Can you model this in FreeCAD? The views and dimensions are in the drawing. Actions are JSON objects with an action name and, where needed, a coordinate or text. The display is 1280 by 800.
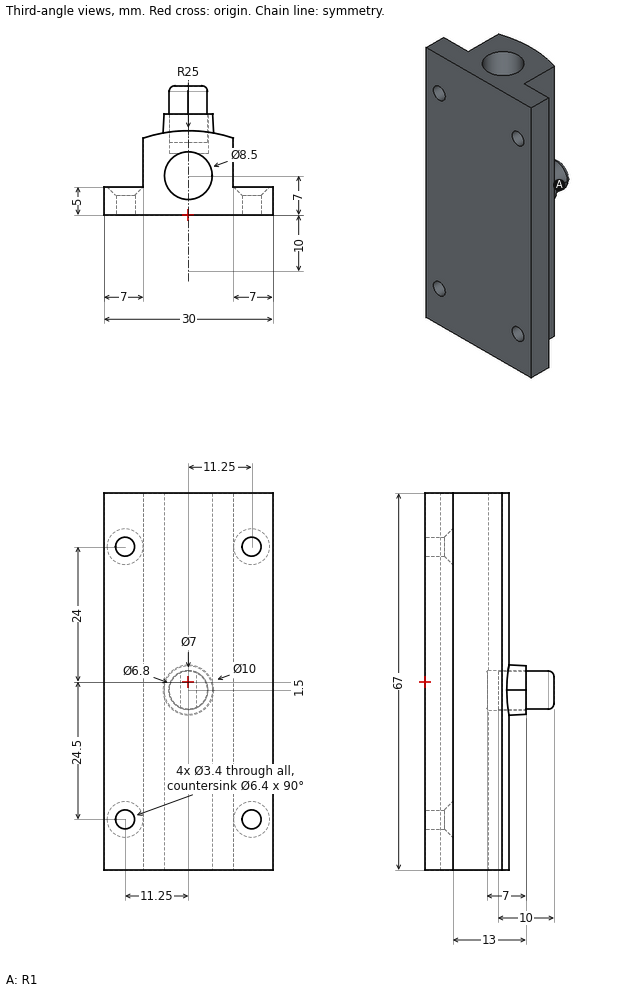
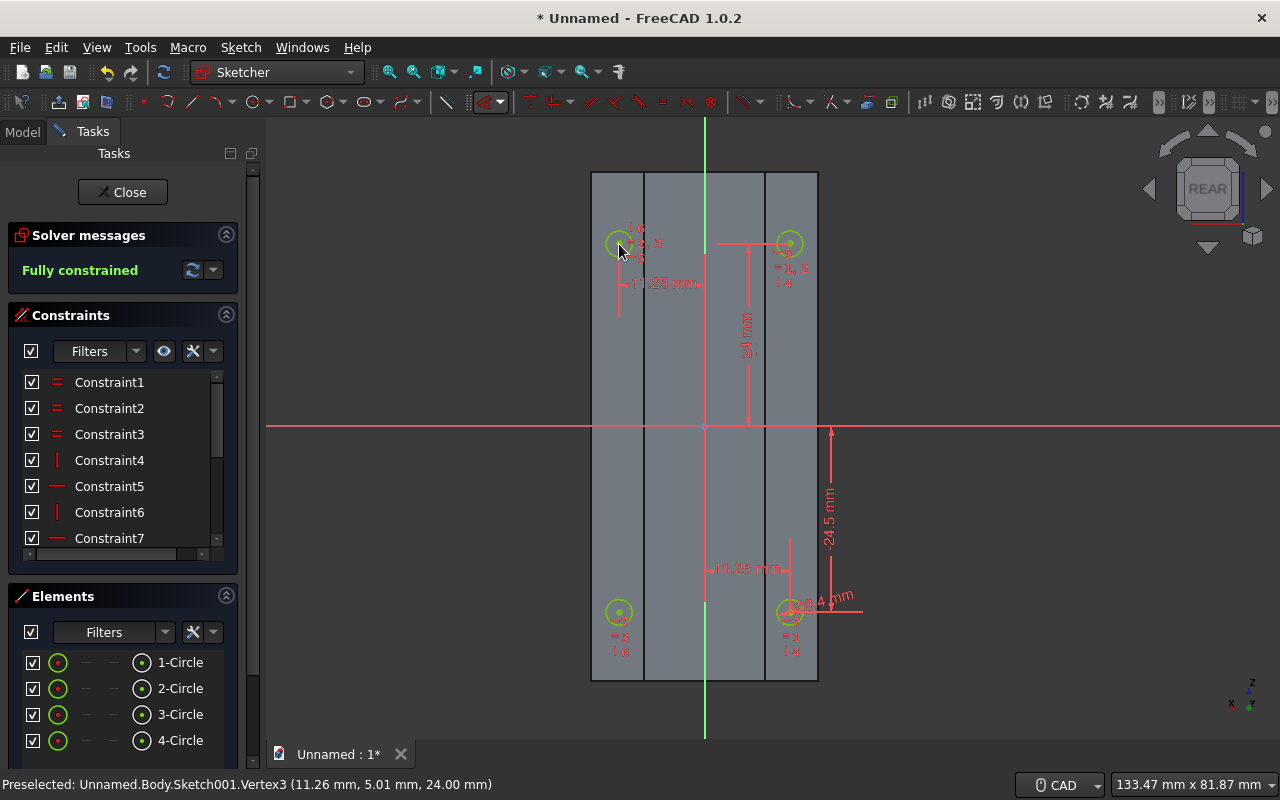
{"action": "left_click", "coordinate": [123, 192]}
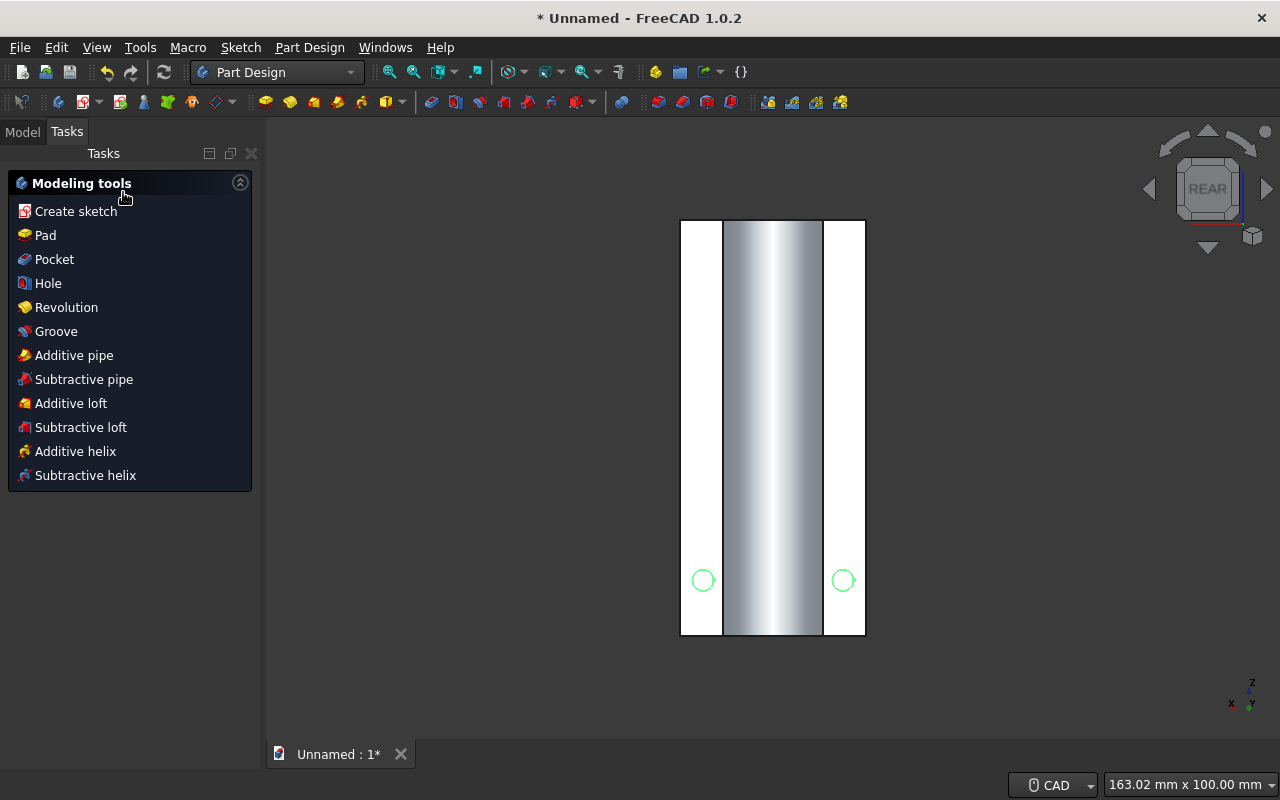
{"action": "left_click", "coordinate": [456, 102]}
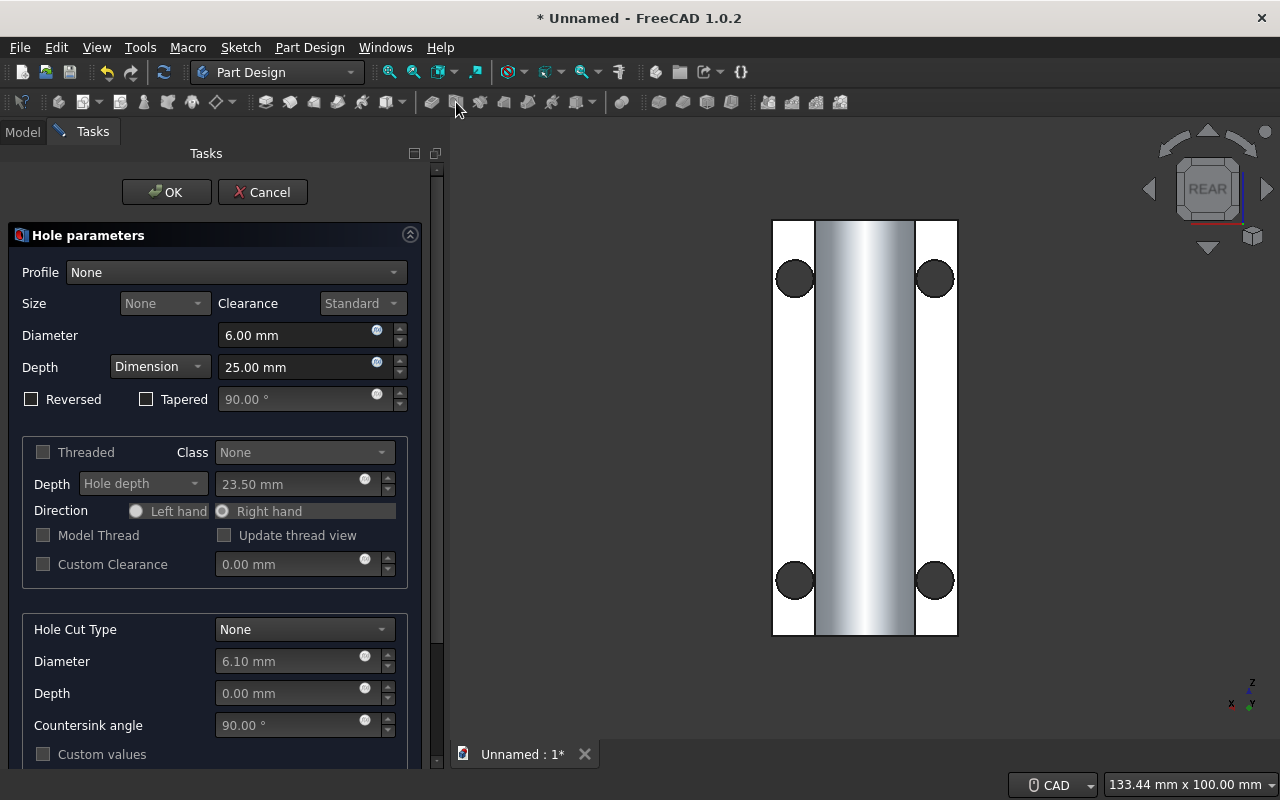
{"action": "triple_click", "coordinate": [305, 335]}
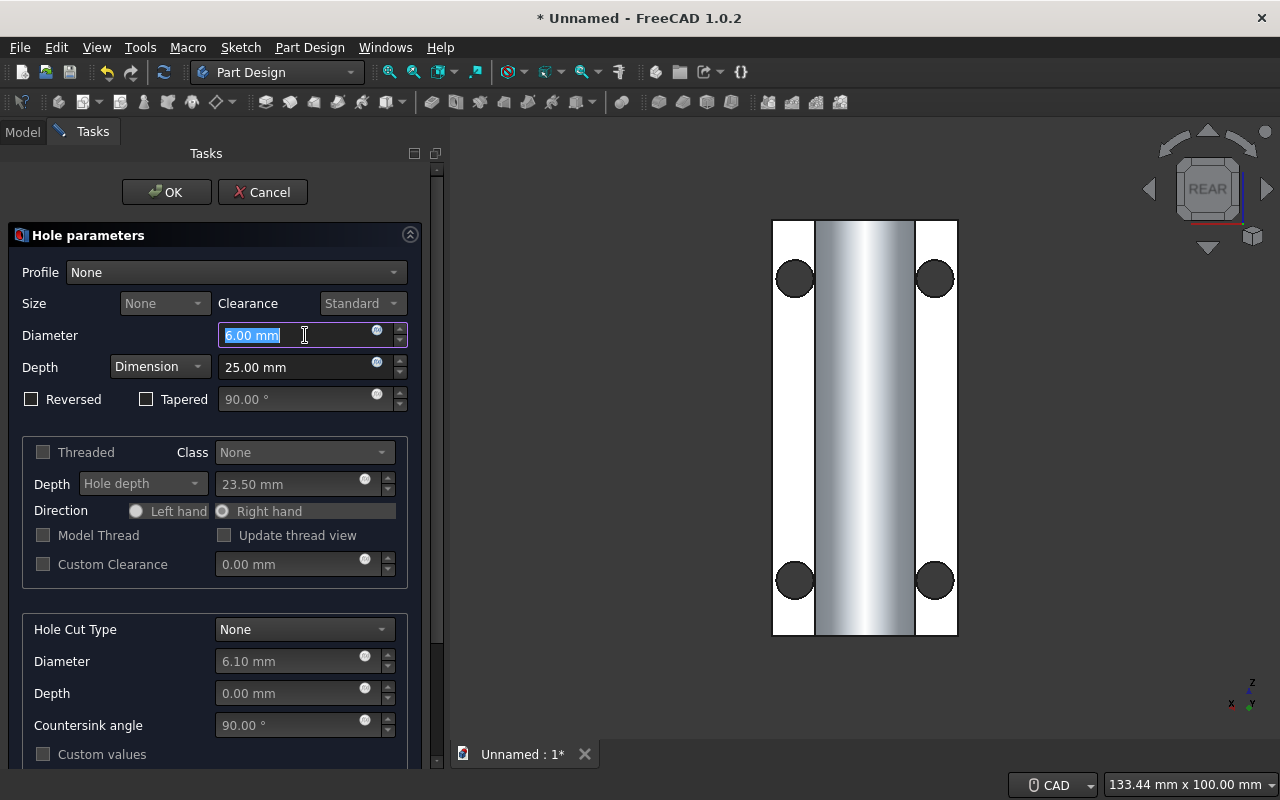
{"action": "type", "text": "3.4"}
{"action": "key", "text": "Tab"}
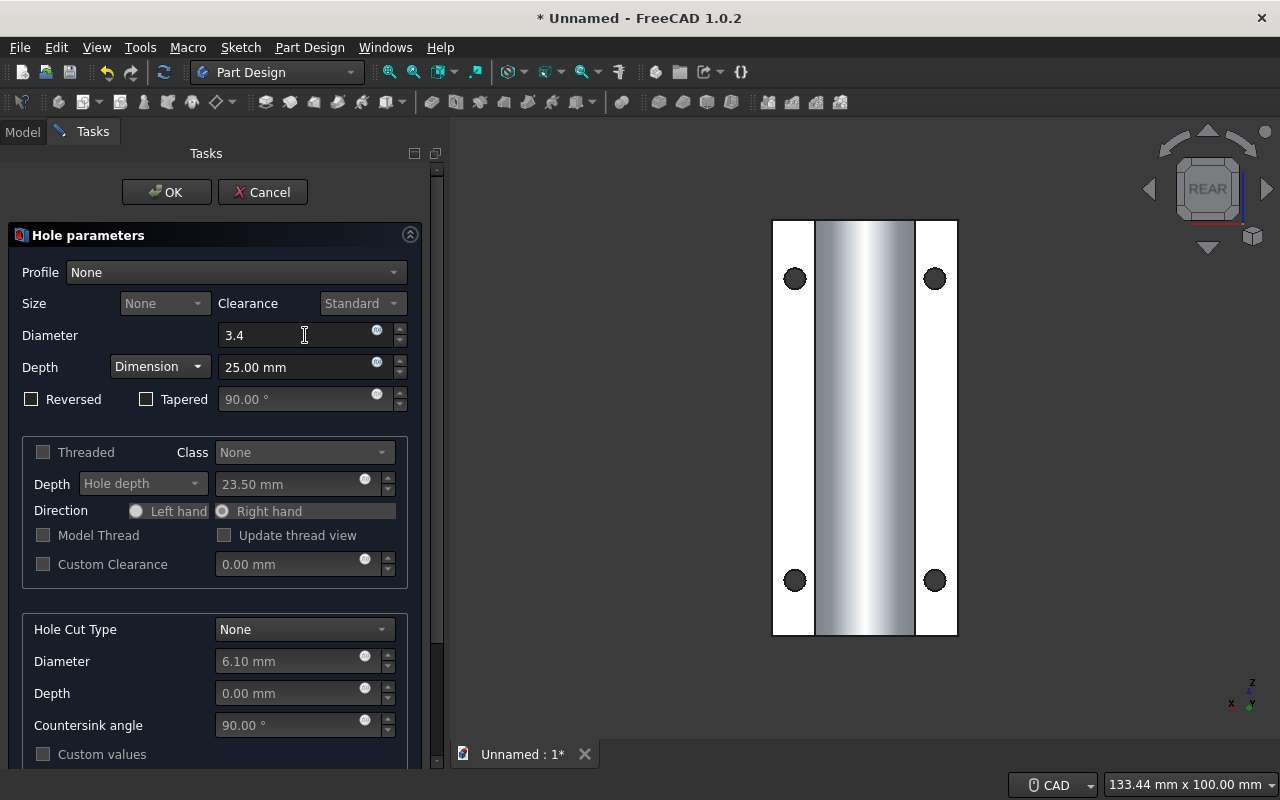
{"action": "left_click", "coordinate": [161, 366]}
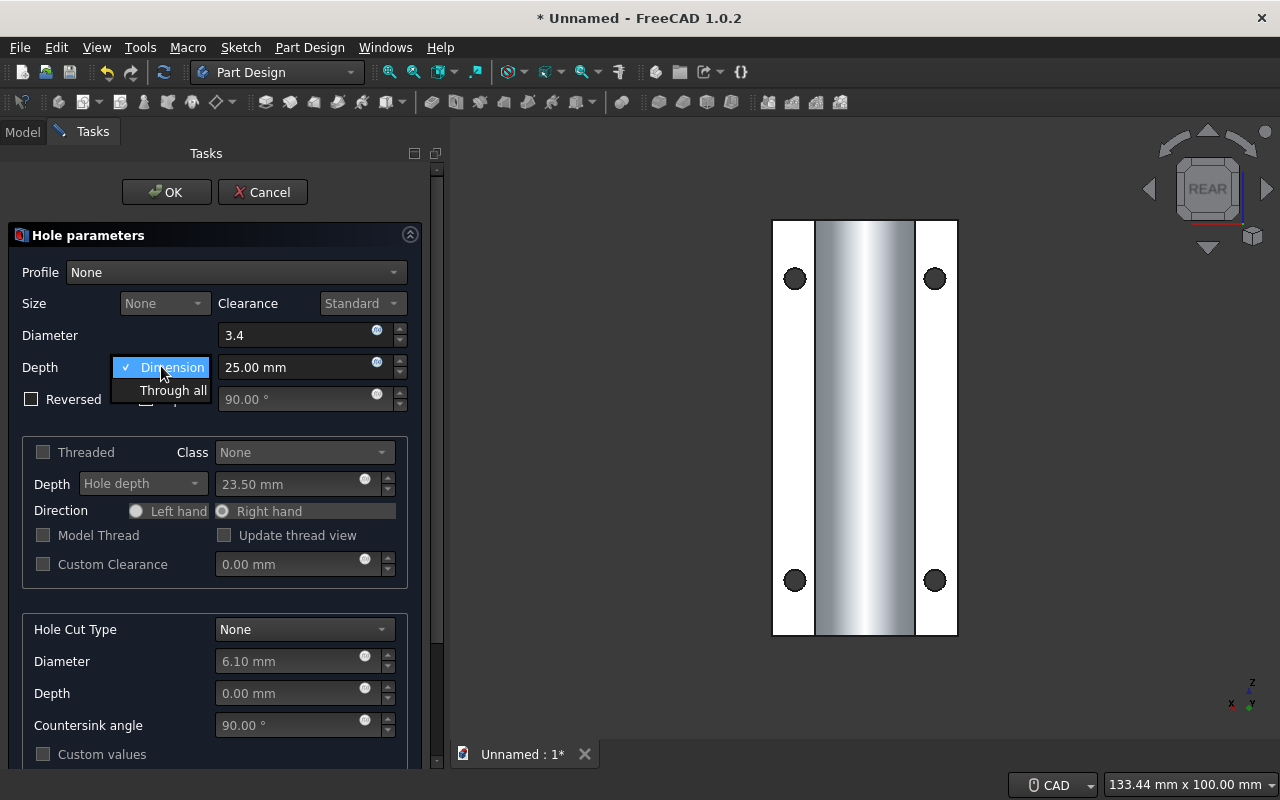
{"action": "left_click", "coordinate": [160, 390]}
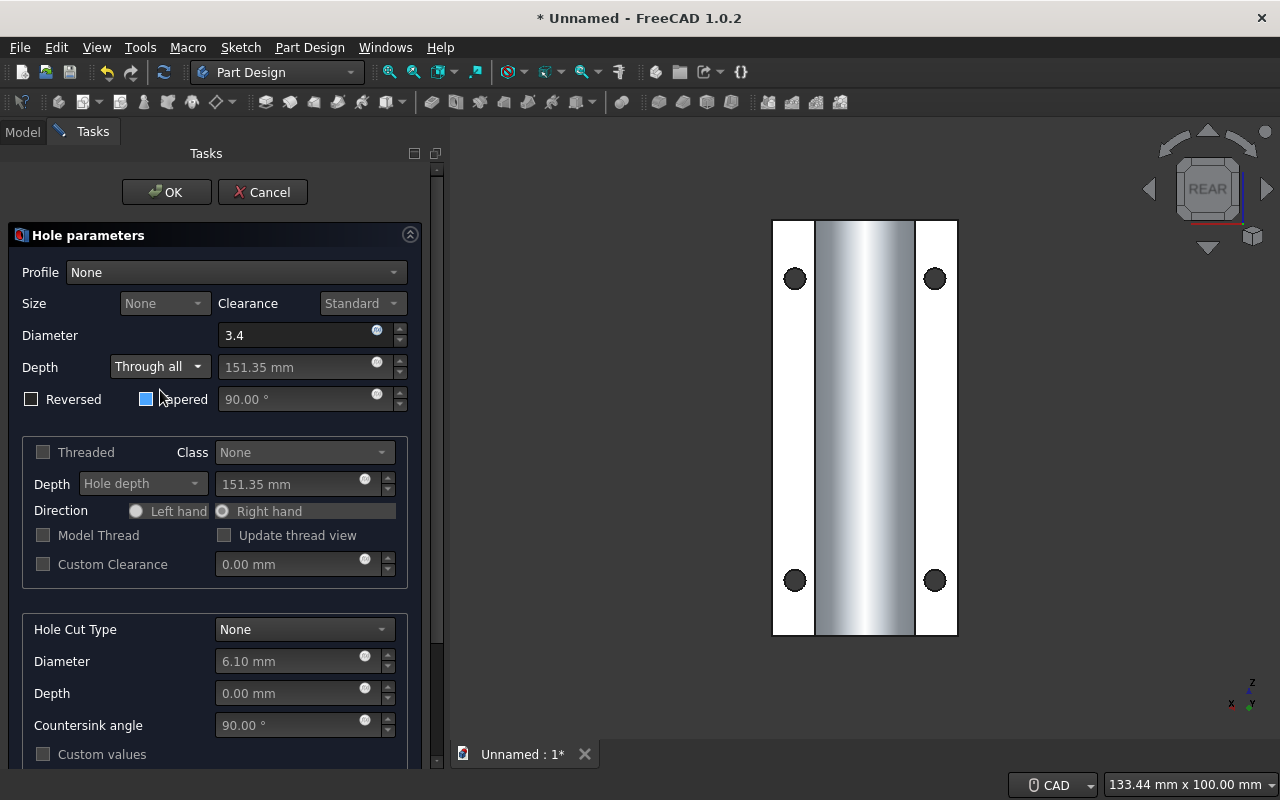
{"action": "left_click", "coordinate": [306, 630]}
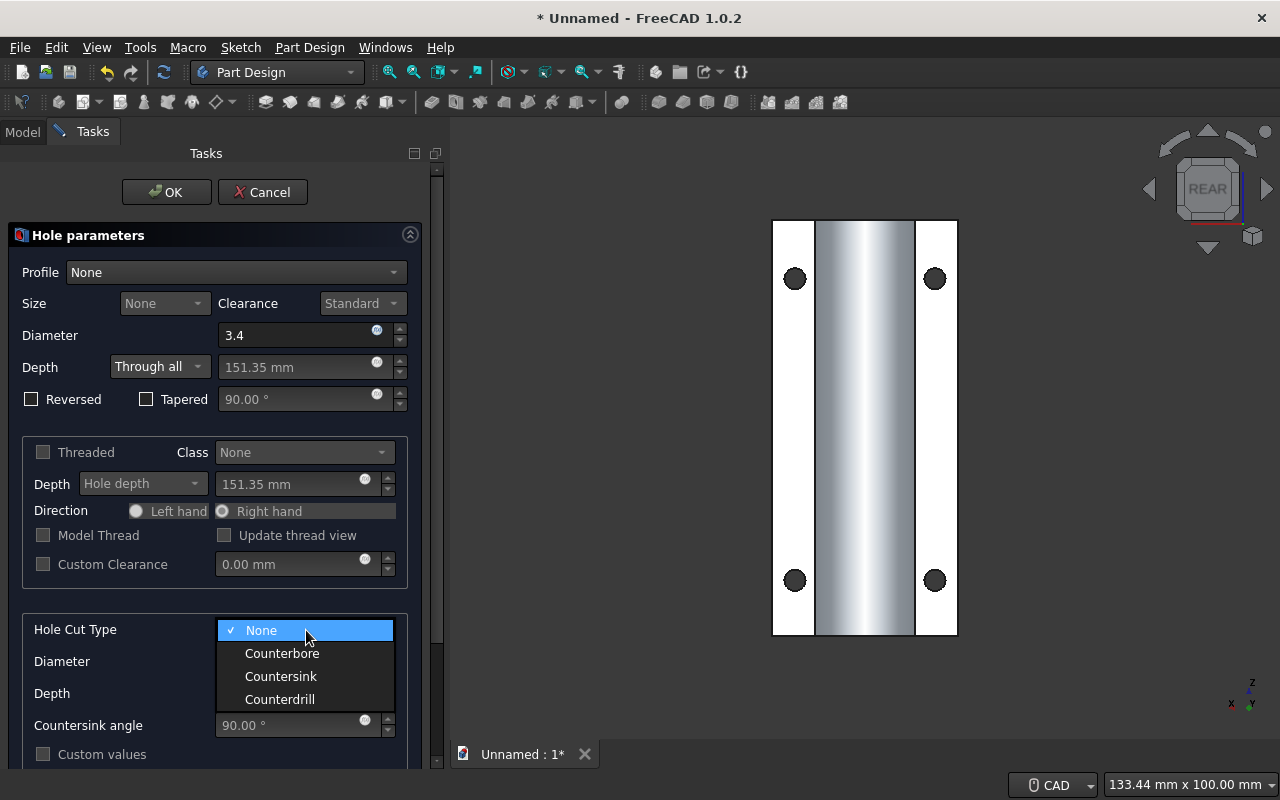
{"action": "left_click", "coordinate": [304, 676]}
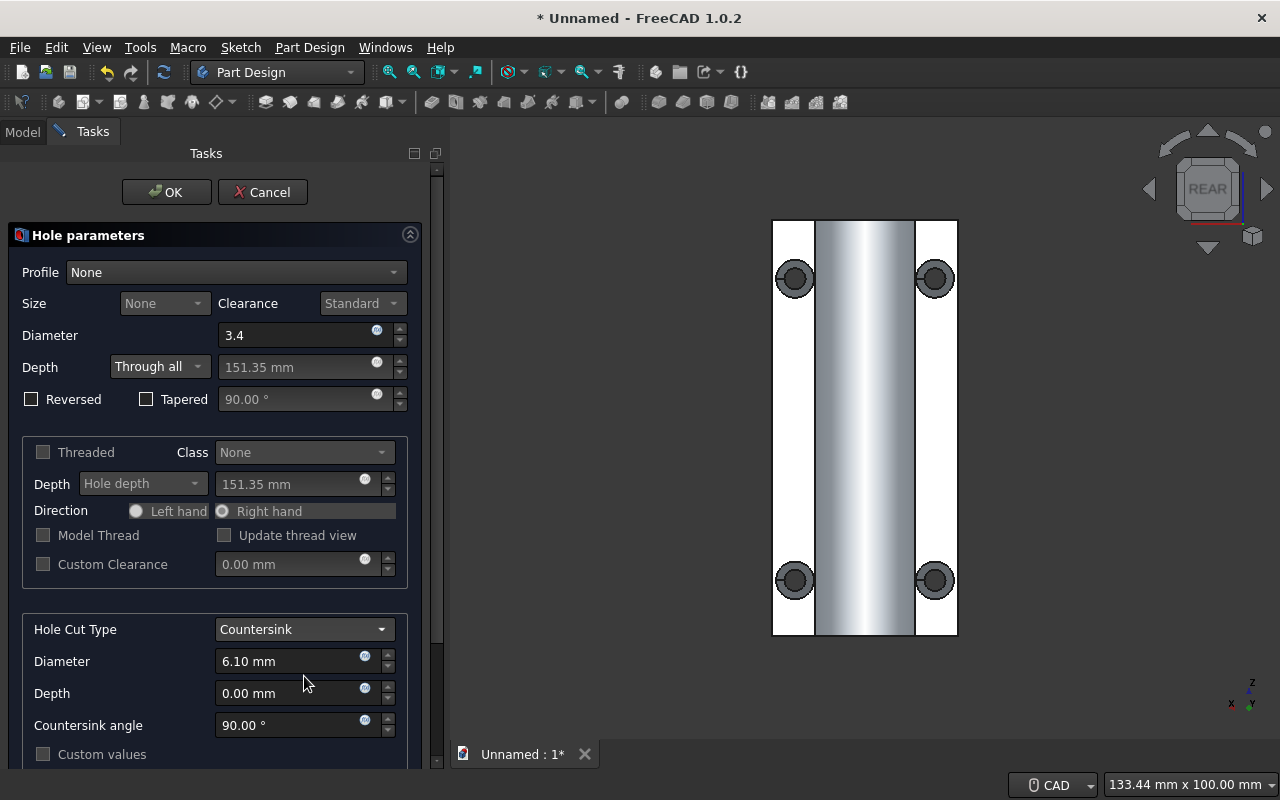
{"action": "triple_click", "coordinate": [298, 661]}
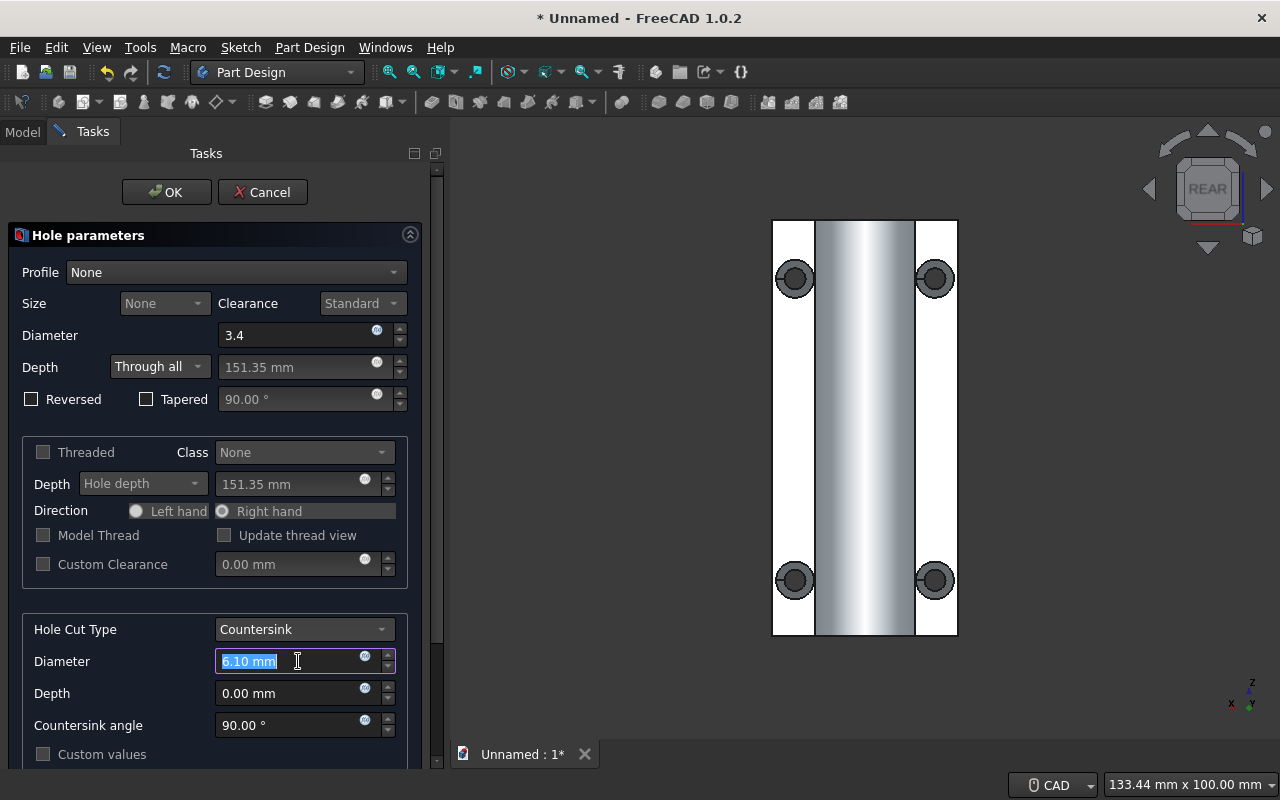
{"action": "type", "text": "6.4"}
{"action": "key", "text": "Tab"}